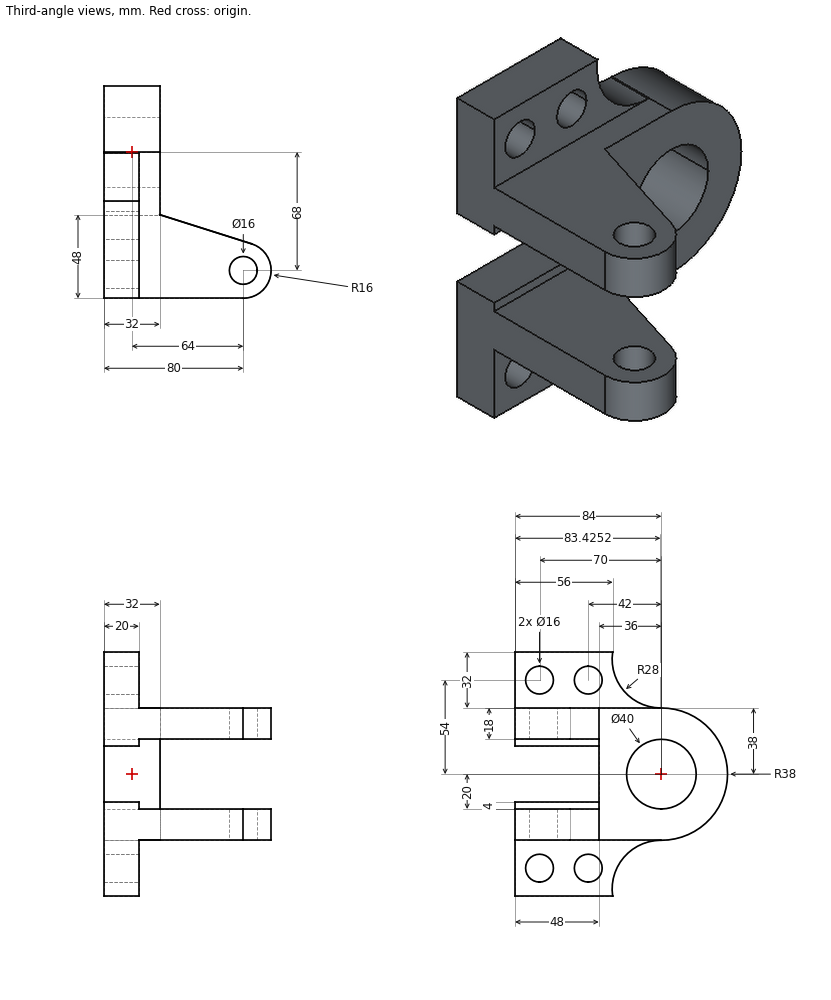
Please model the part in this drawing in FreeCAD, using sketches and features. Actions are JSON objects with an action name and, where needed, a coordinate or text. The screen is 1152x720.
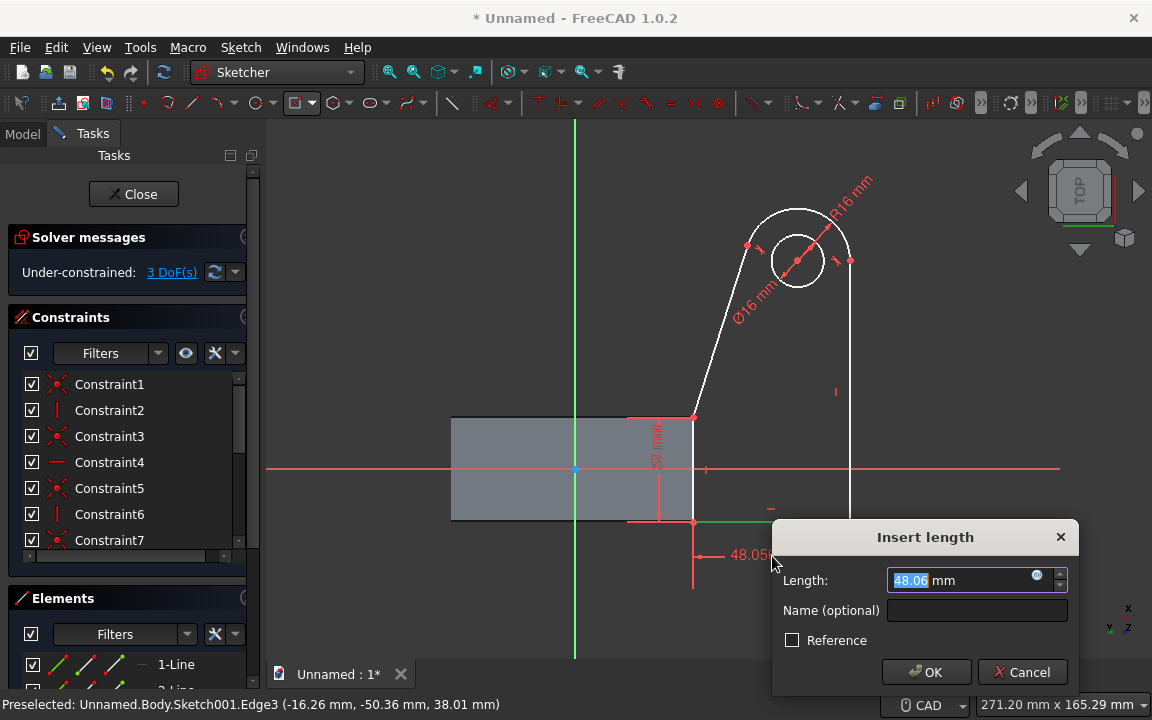
{"action": "type", "text": "48"}
{"action": "key", "text": "Return"}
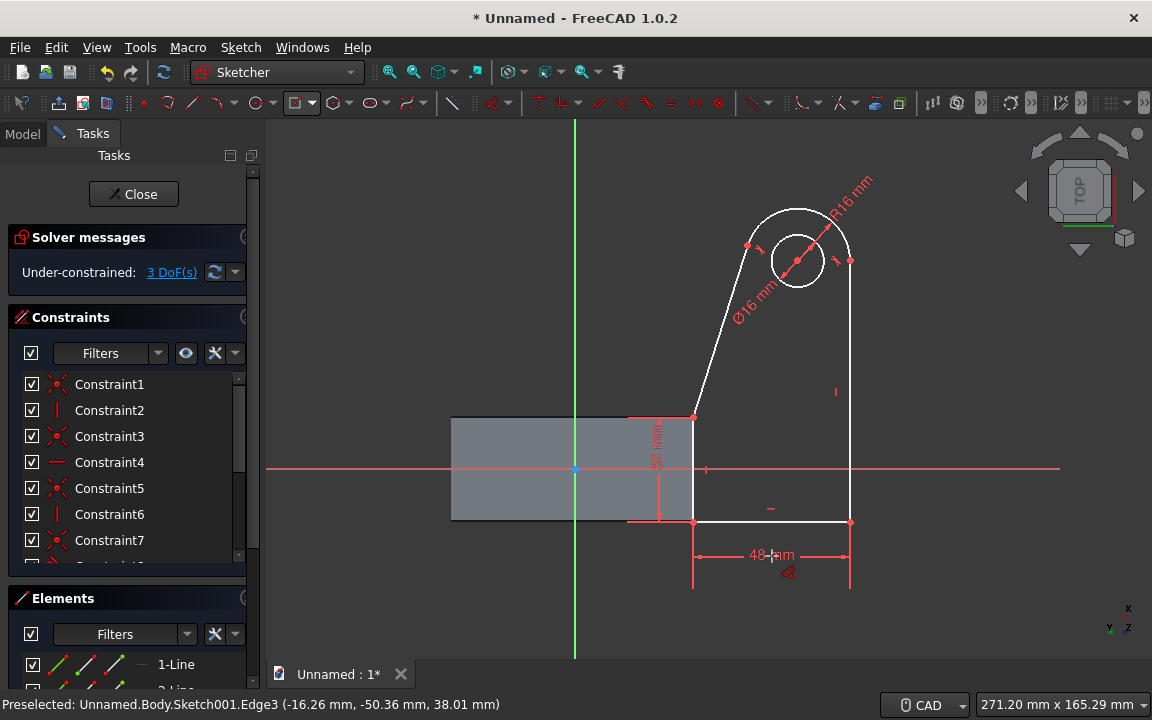
{"action": "left_click", "coordinate": [850, 444]}
{"action": "left_click", "coordinate": [884, 392]}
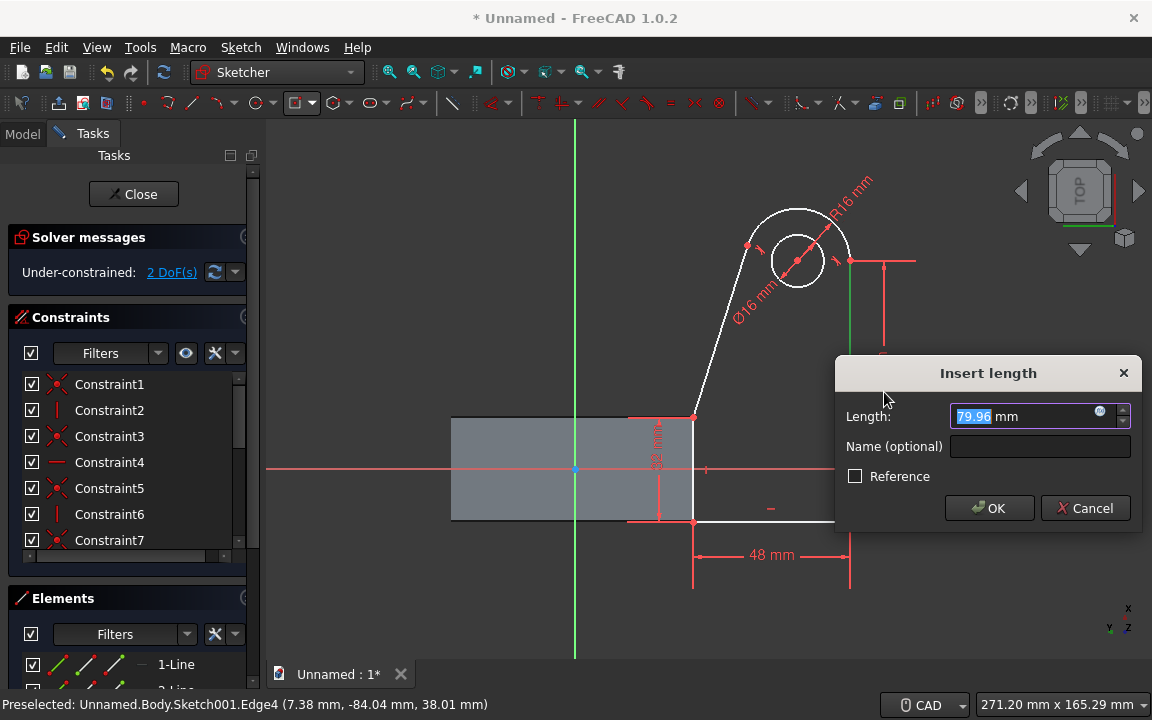
{"action": "type", "text": "80"}
{"action": "key", "text": "Return"}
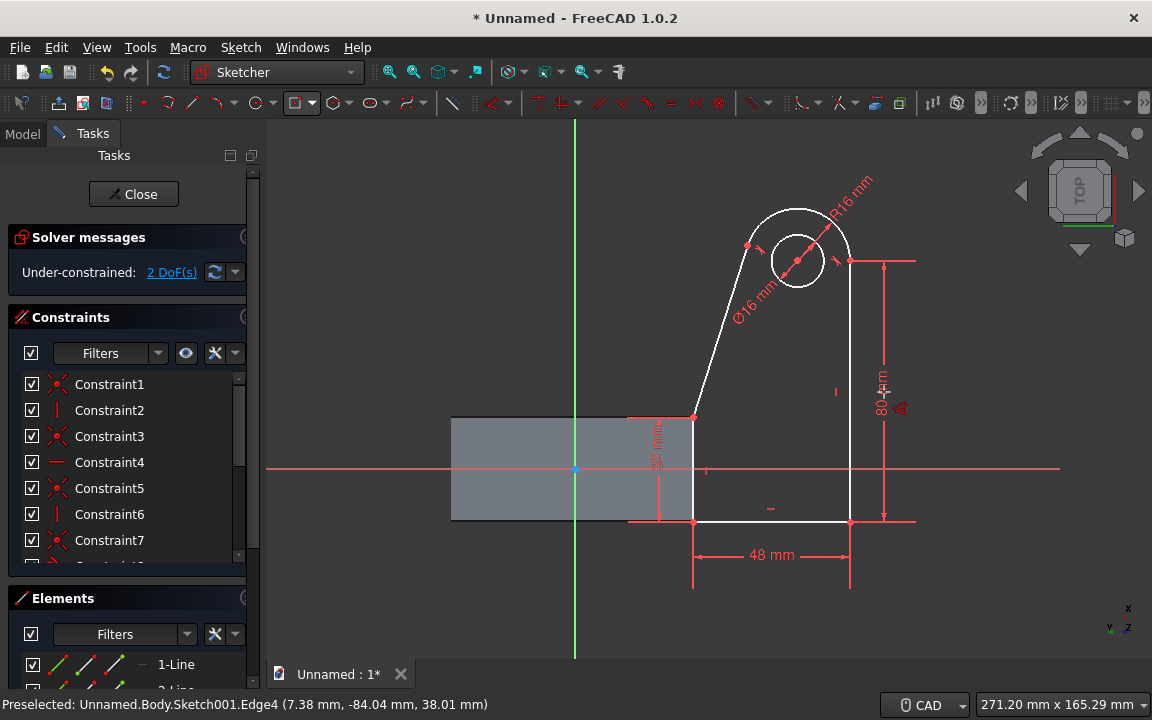
{"action": "left_click", "coordinate": [798, 261]}
{"action": "left_click", "coordinate": [635, 503]}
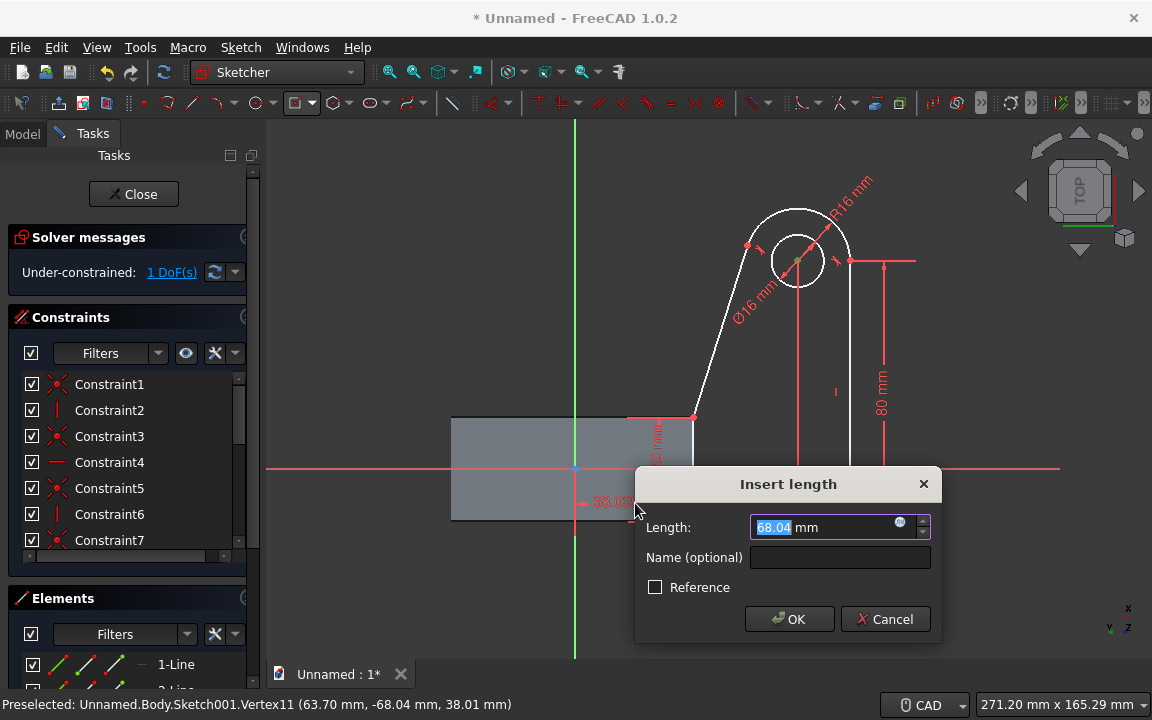
{"action": "type", "text": "68"}
{"action": "key", "text": "Return"}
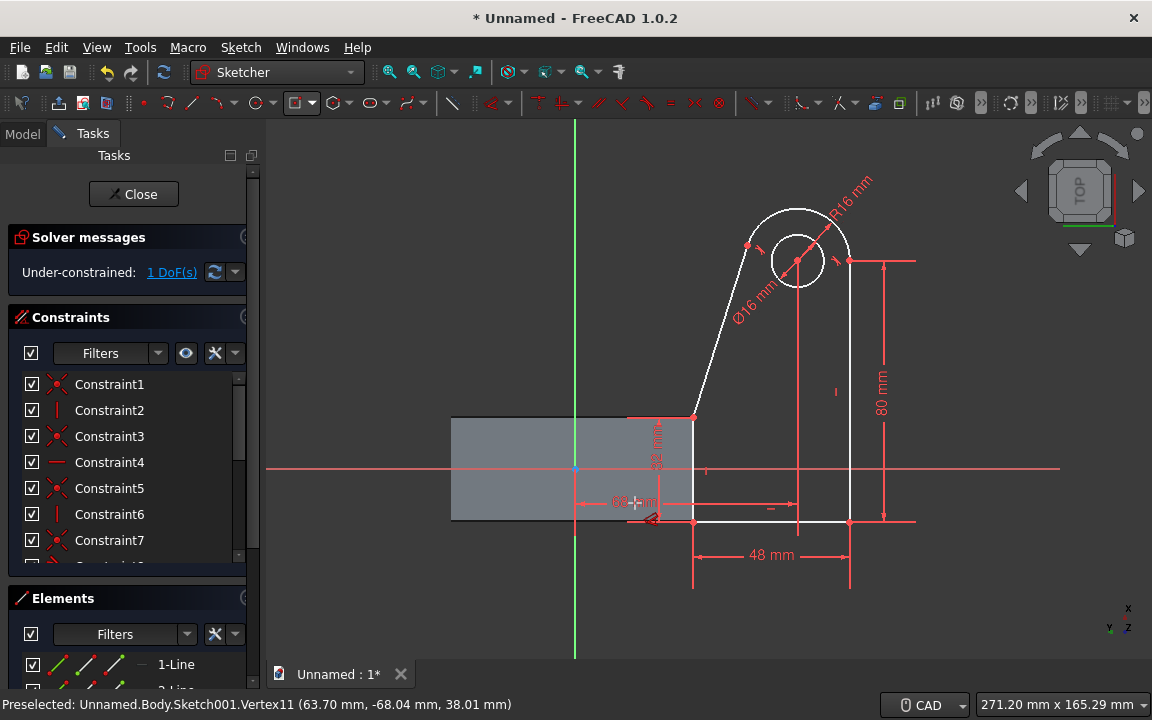
{"action": "left_click", "coordinate": [798, 261]}
{"action": "left_click", "coordinate": [541, 365]}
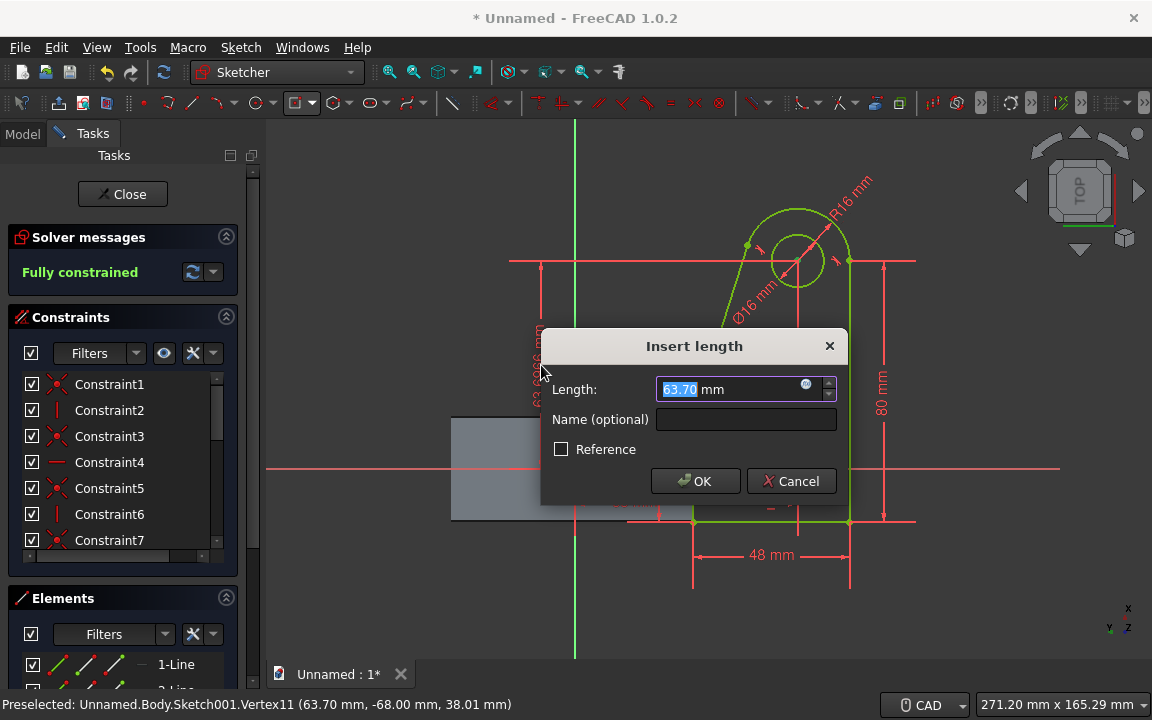
{"action": "type", "text": "64"}
{"action": "key", "text": "Return"}
{"action": "key", "text": "Escape"}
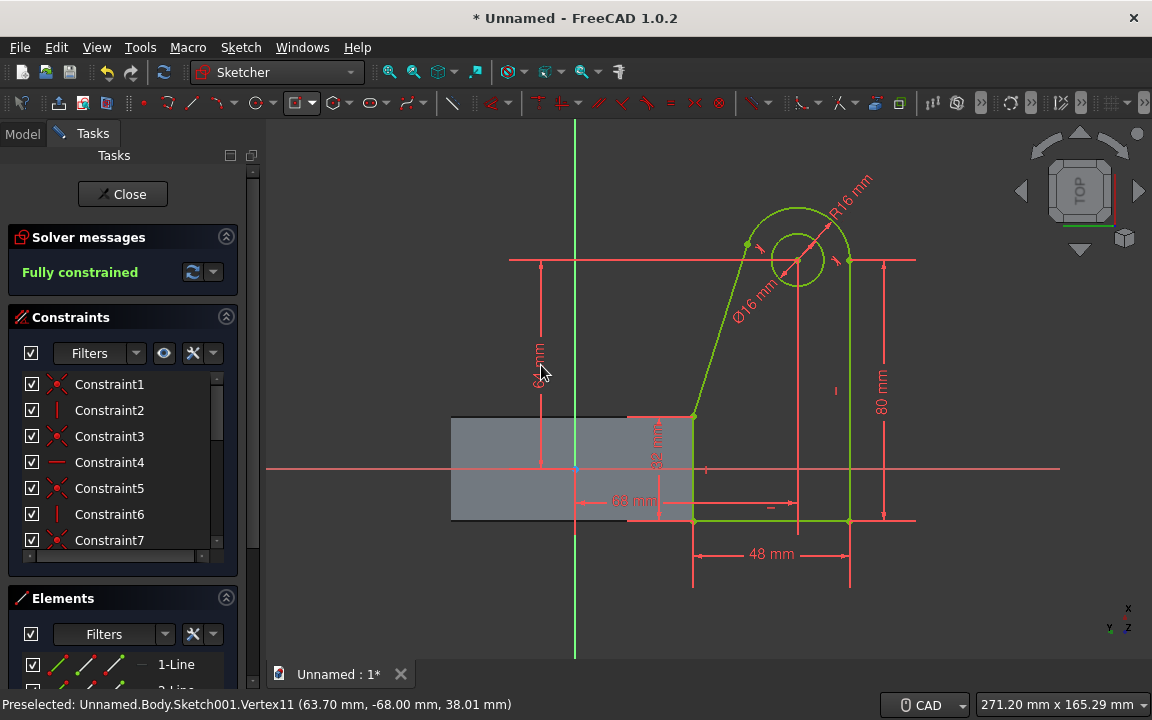
{"action": "left_click", "coordinate": [123, 194]}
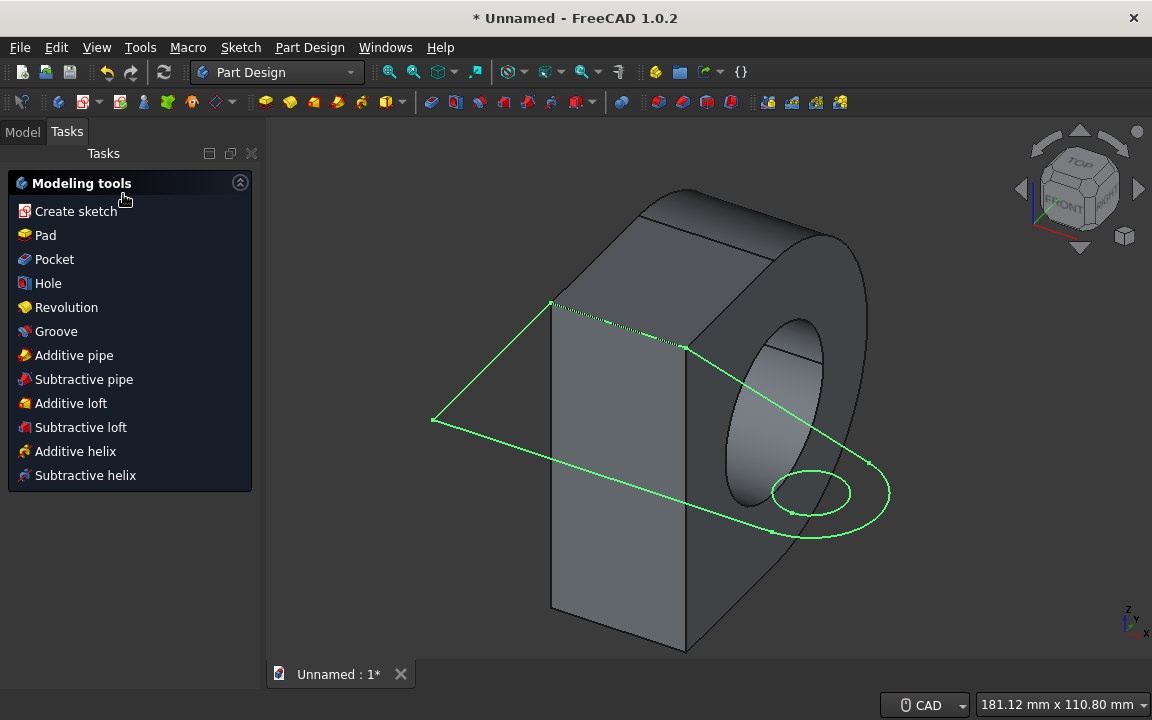
{"action": "left_click", "coordinate": [266, 102]}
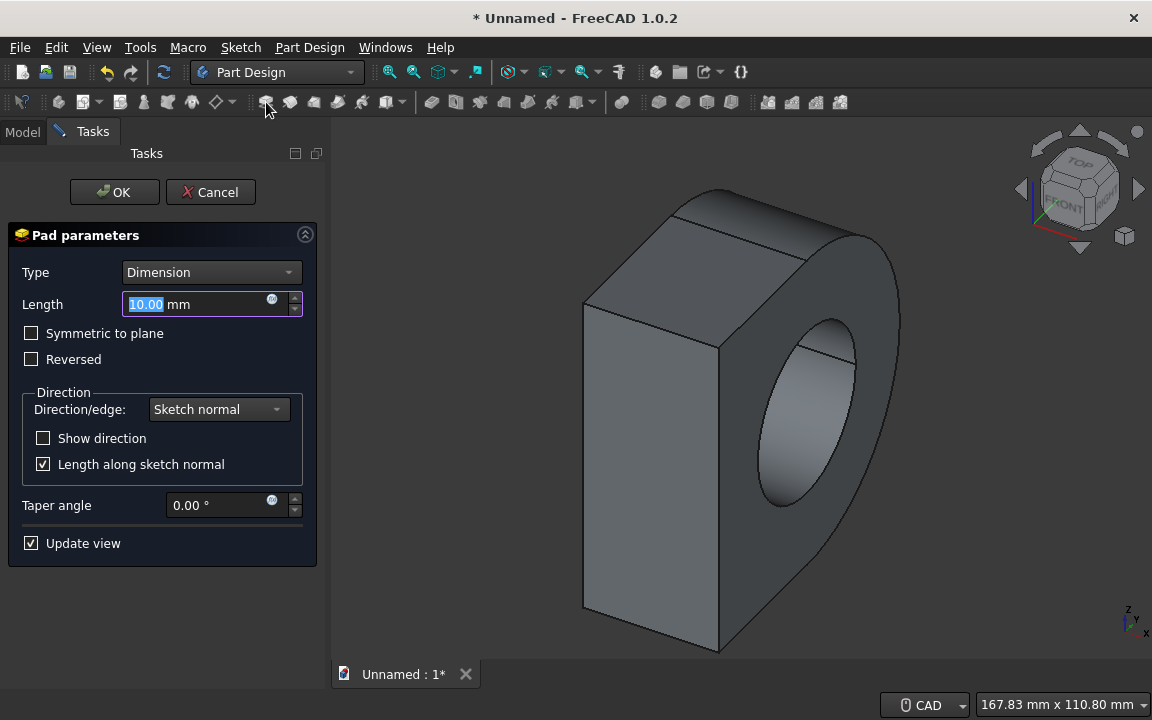
{"action": "type", "text": "18"}
{"action": "key", "text": "Tab"}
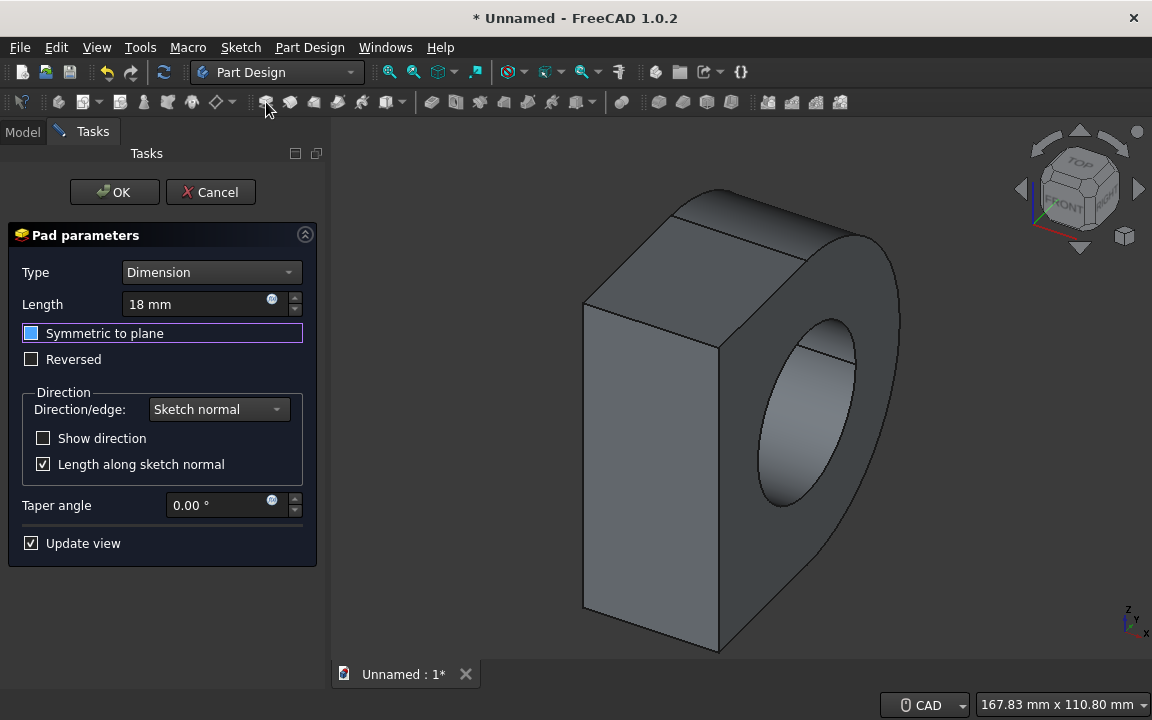
{"action": "left_click", "coordinate": [30, 359]}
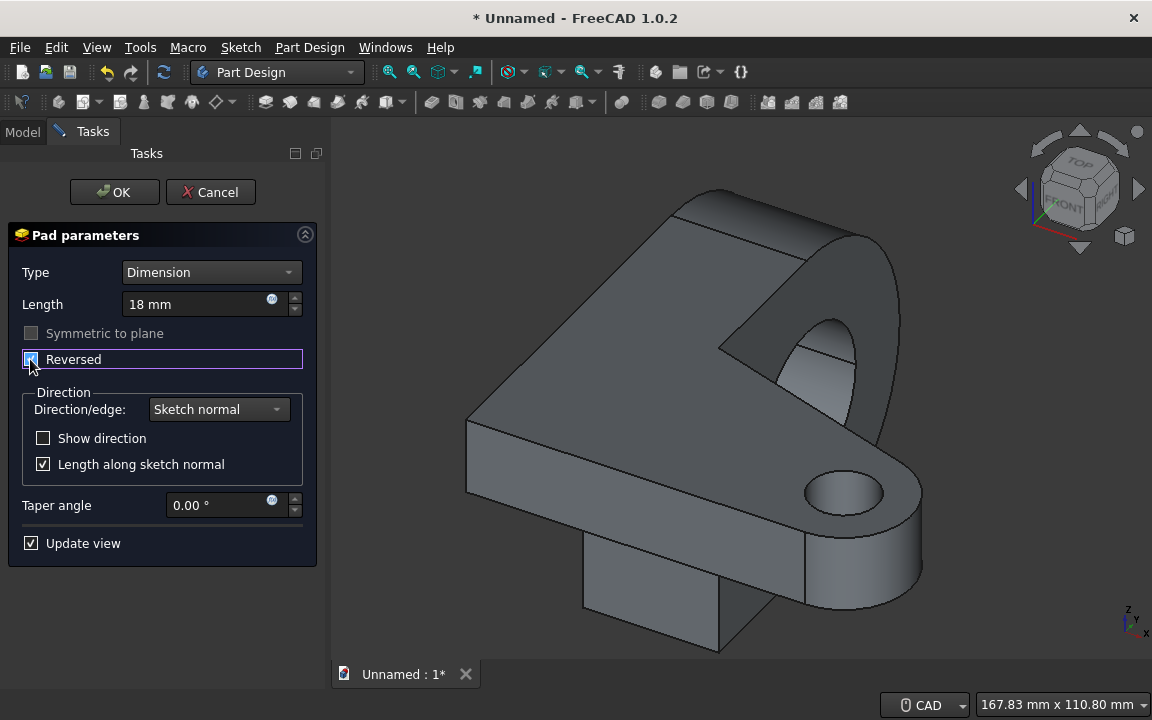
{"action": "left_click", "coordinate": [115, 192]}